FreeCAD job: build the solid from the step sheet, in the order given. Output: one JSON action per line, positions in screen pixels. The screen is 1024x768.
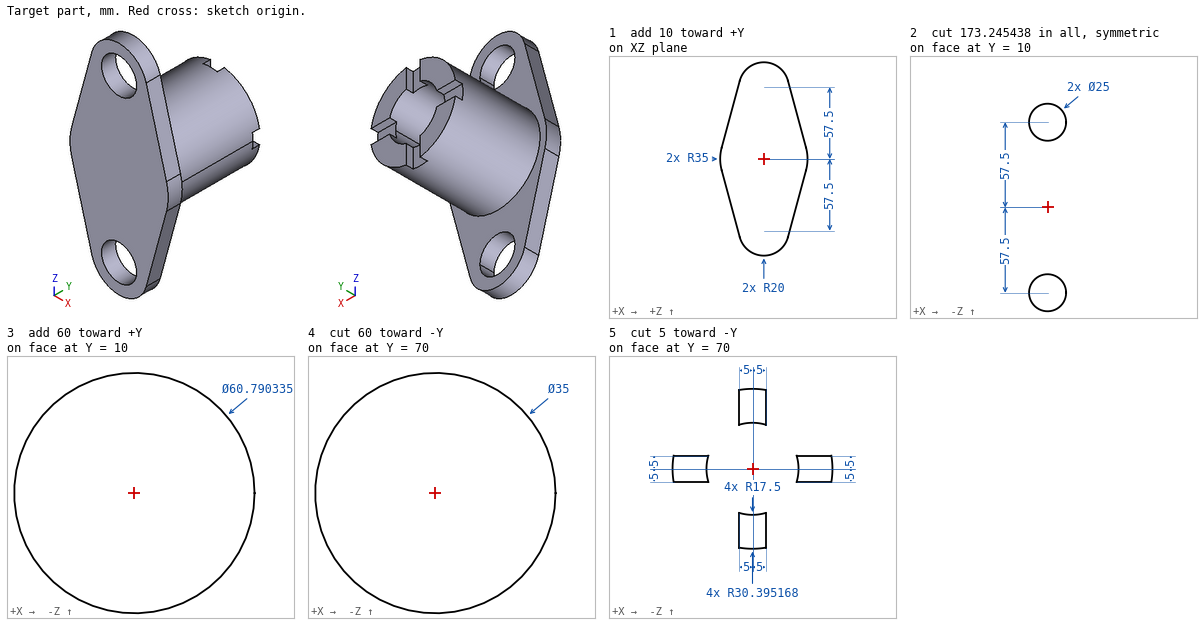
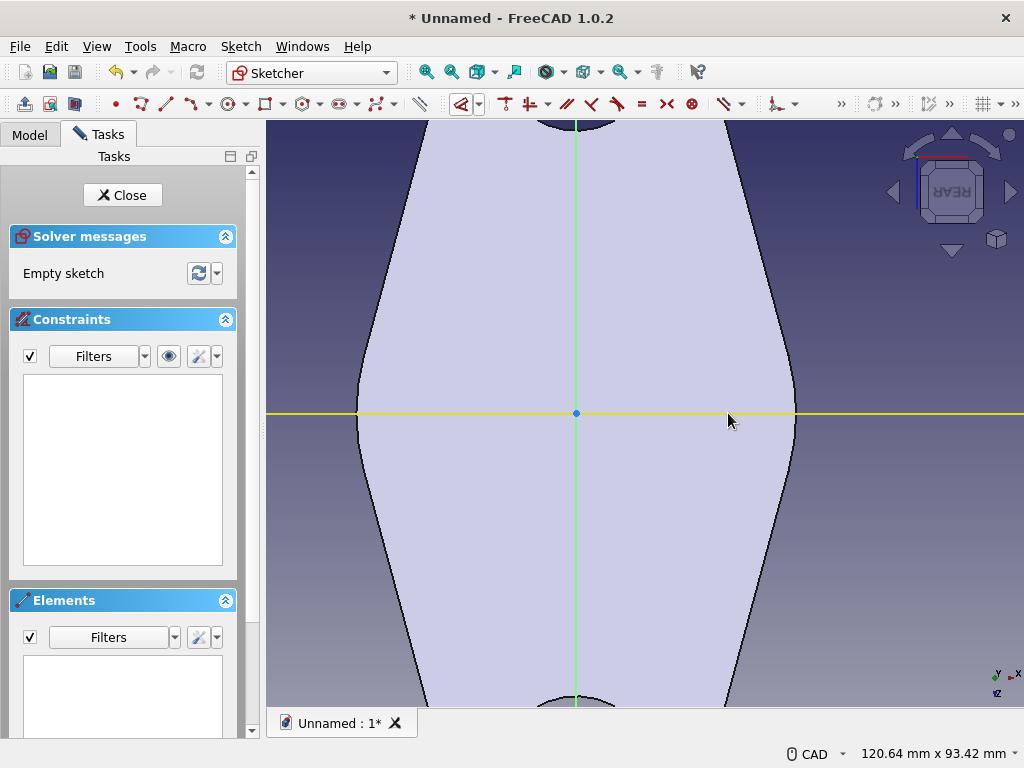
{"action": "left_click", "coordinate": [228, 104]}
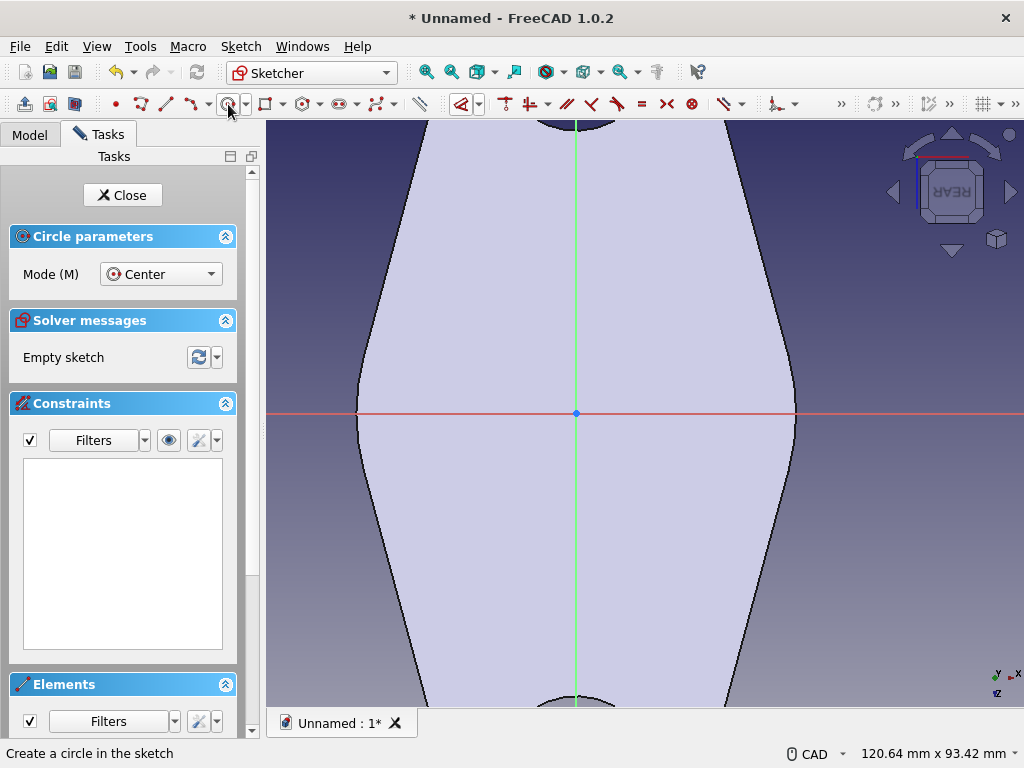
{"action": "left_click", "coordinate": [576, 413]}
{"action": "mouse_move", "coordinate": [711, 278]}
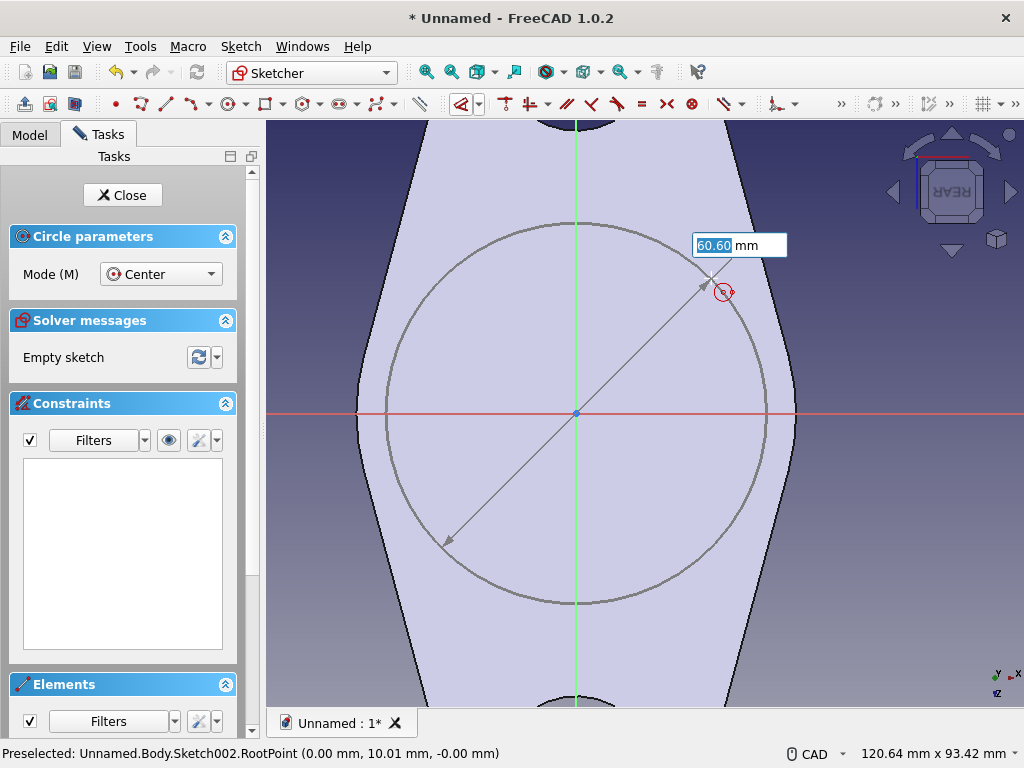
{"action": "type", "text": "60.790335"}
{"action": "key", "text": "Return"}
{"action": "key", "text": "Escape"}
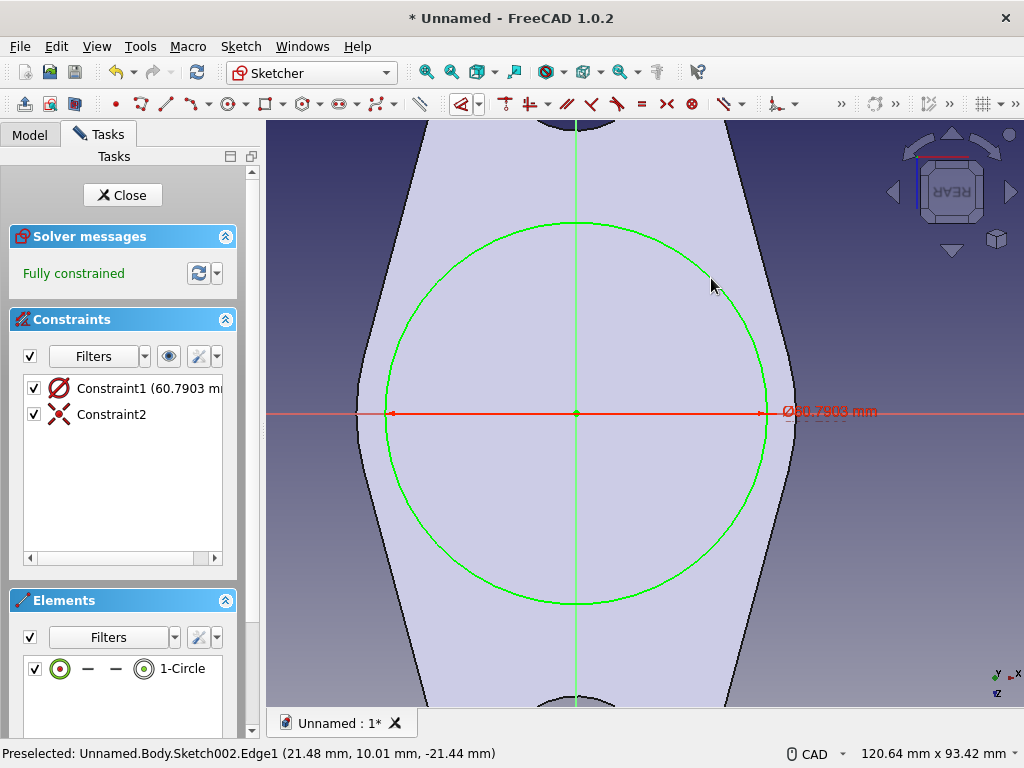
{"action": "left_click", "coordinate": [123, 195]}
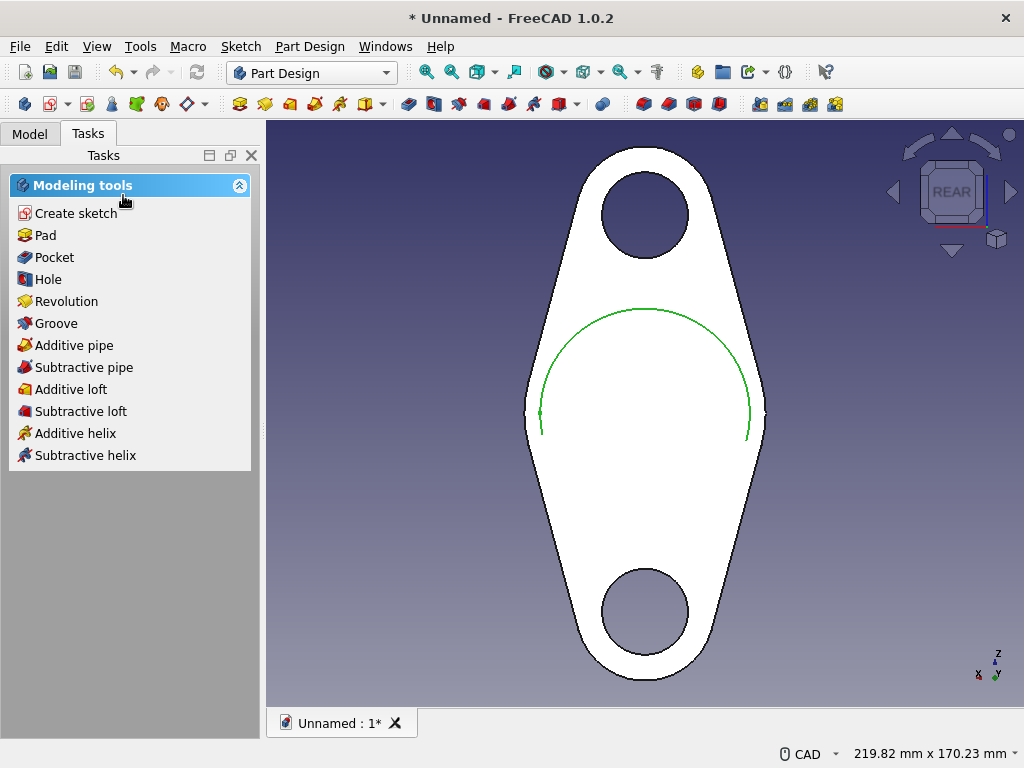
{"action": "left_click", "coordinate": [240, 104]}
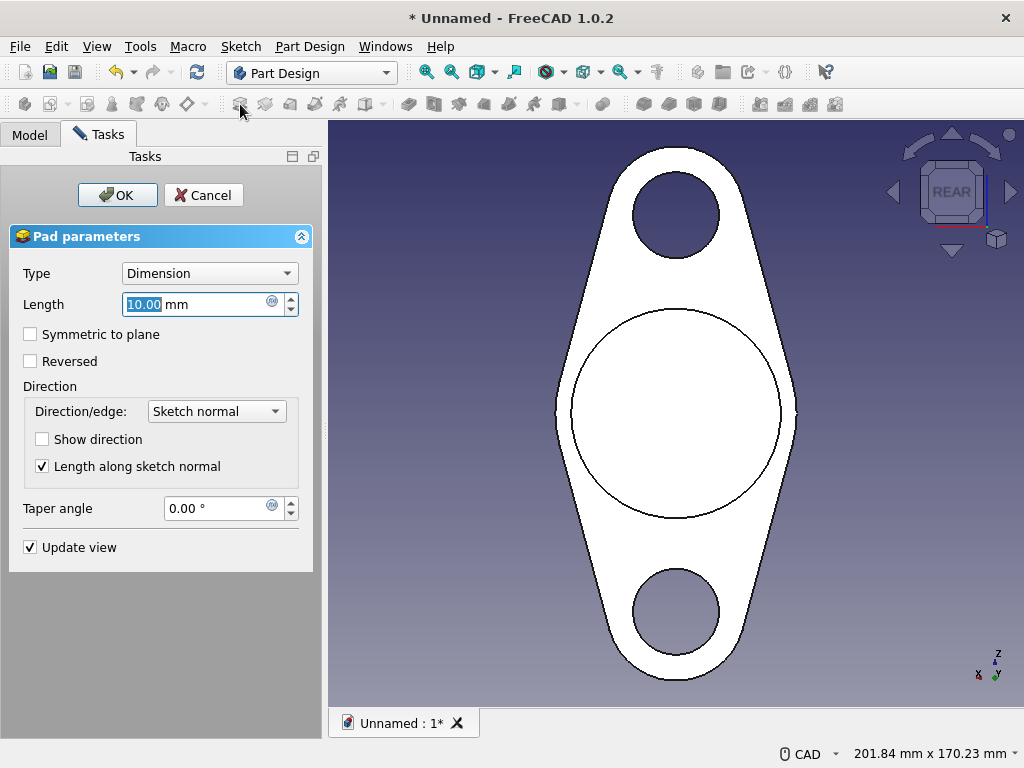
{"action": "type", "text": "60"}
{"action": "key", "text": "Tab"}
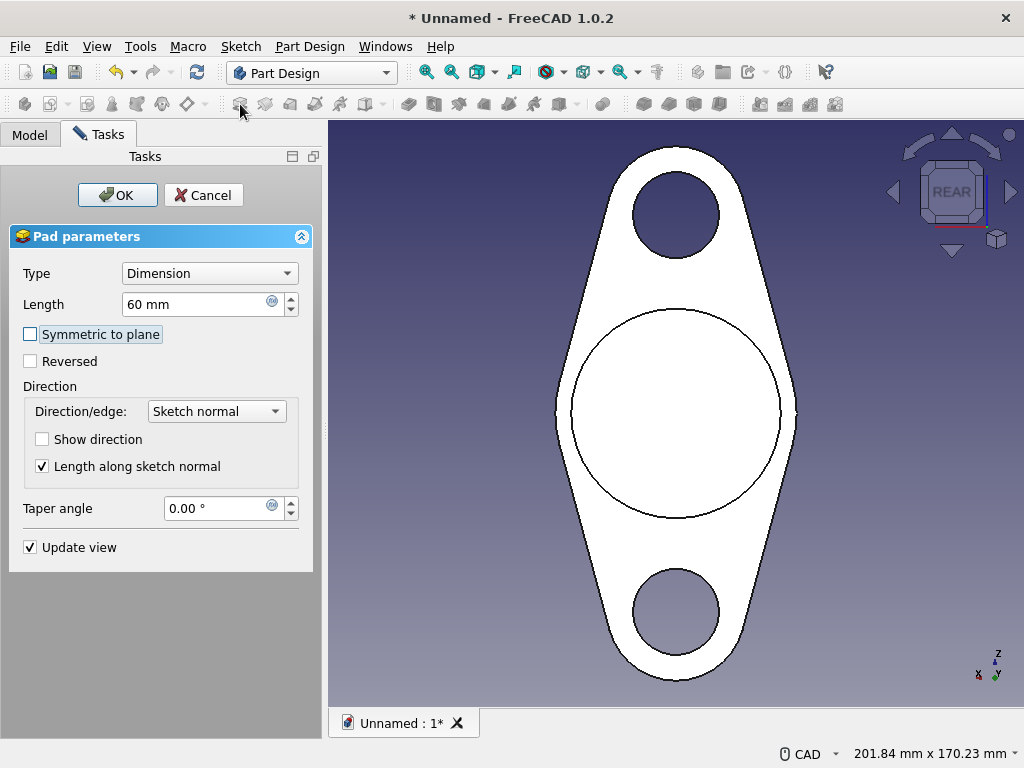
{"action": "left_click", "coordinate": [118, 195]}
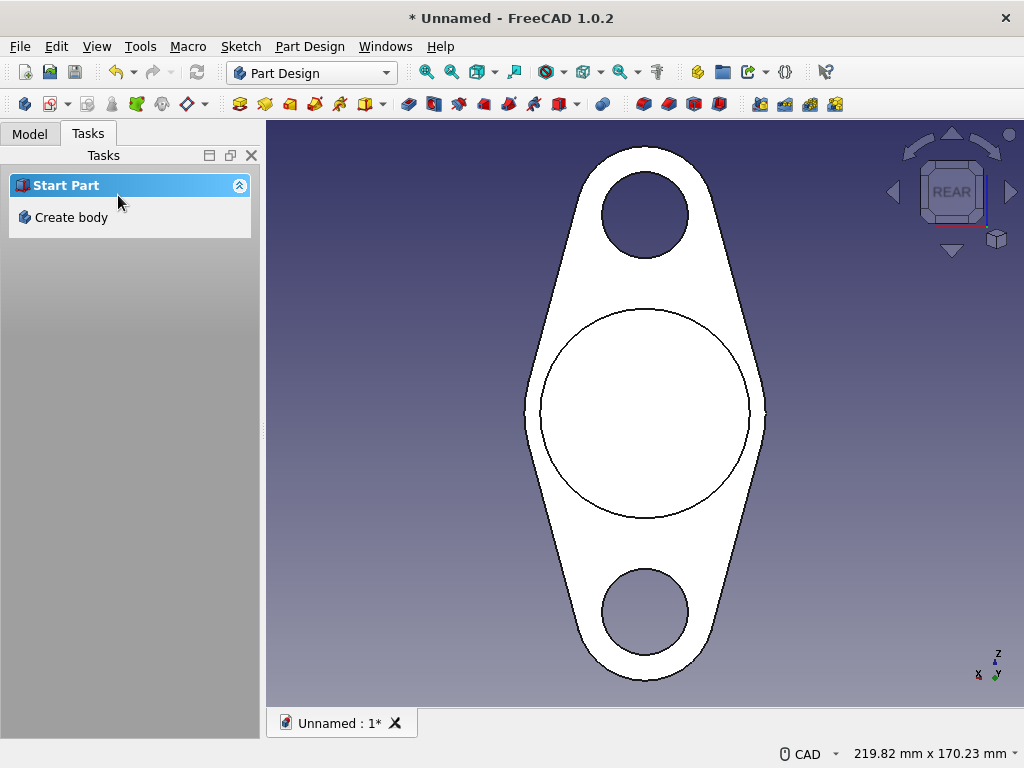
{"action": "left_click", "coordinate": [645, 412]}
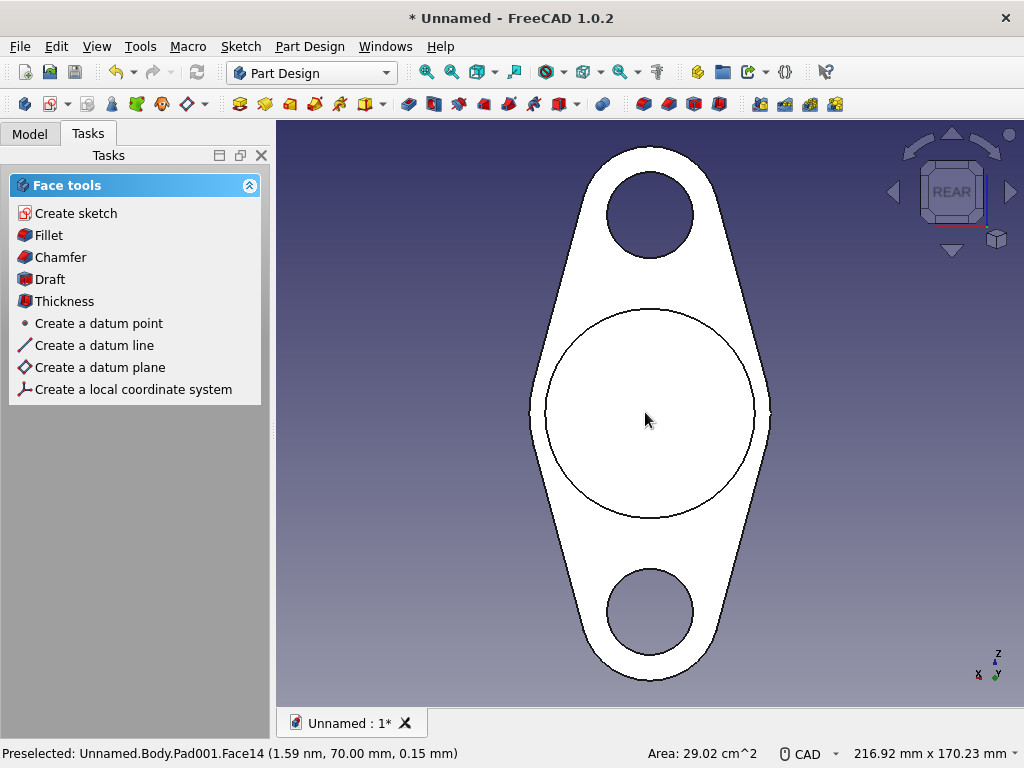
{"action": "left_click", "coordinate": [50, 104]}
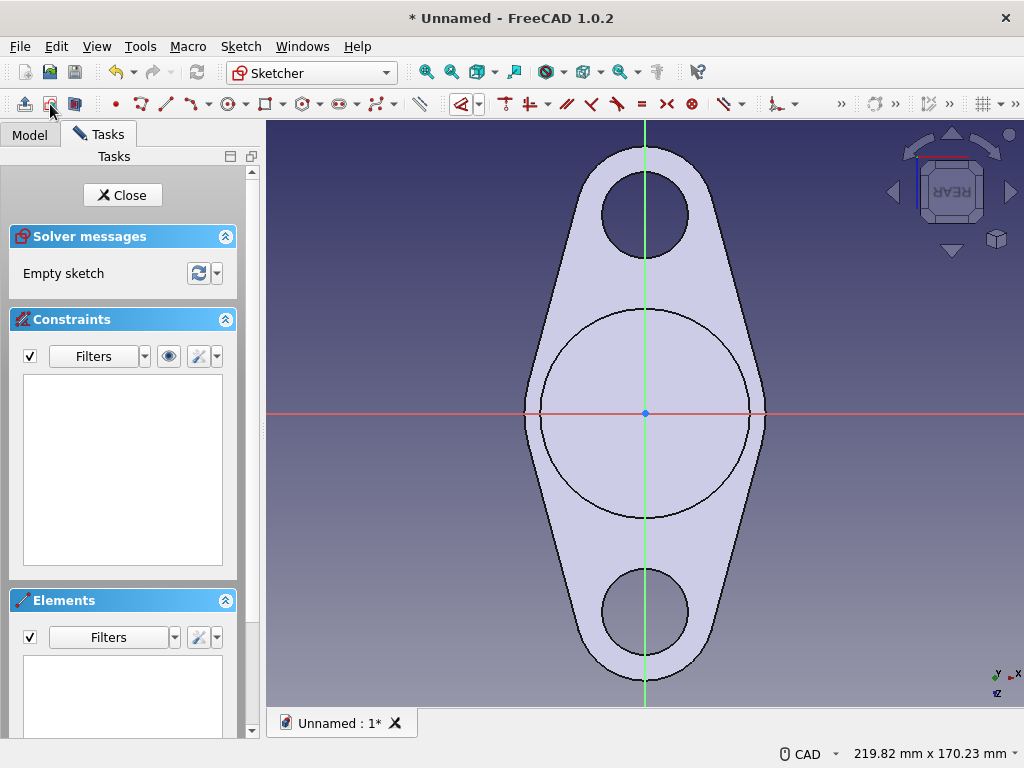
{"action": "scroll", "coordinate": [675, 413], "scroll_direction": "up", "scroll_amount": 6}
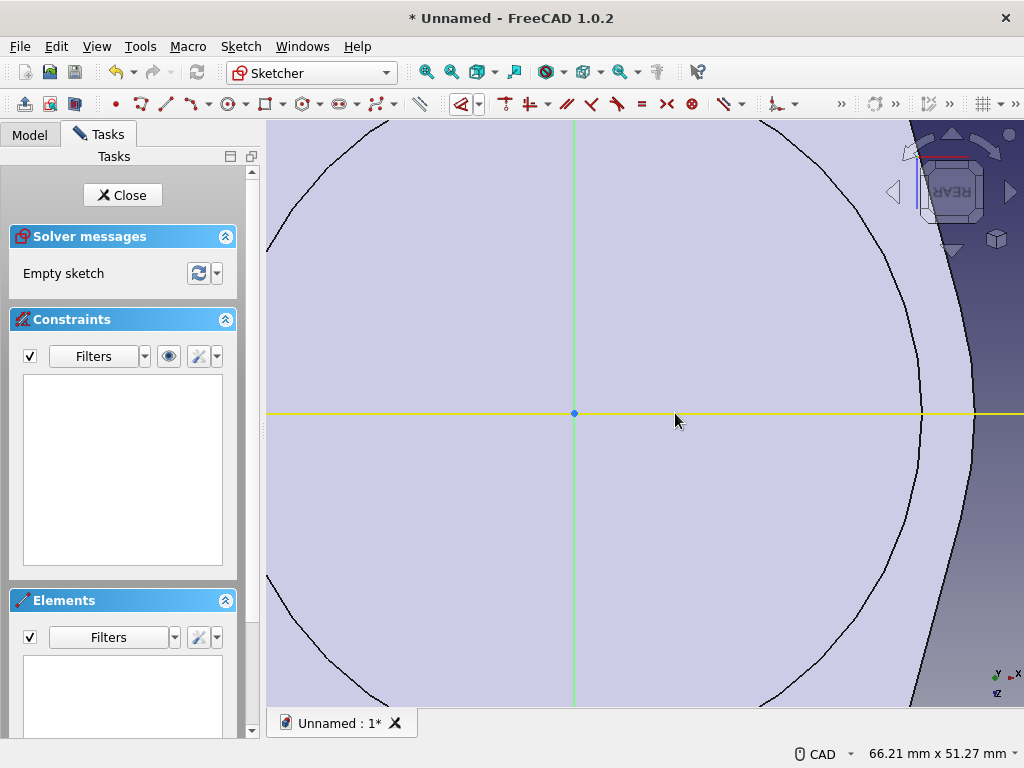
{"action": "left_click", "coordinate": [228, 104]}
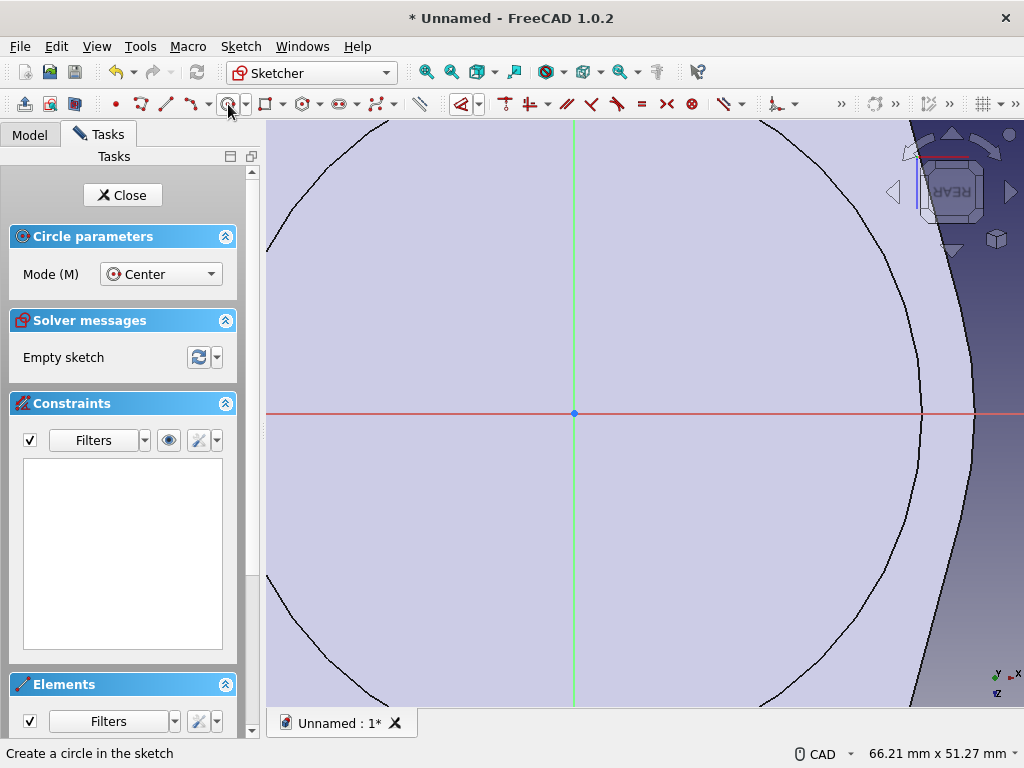
{"action": "left_click", "coordinate": [574, 413]}
{"action": "mouse_move", "coordinate": [716, 272]}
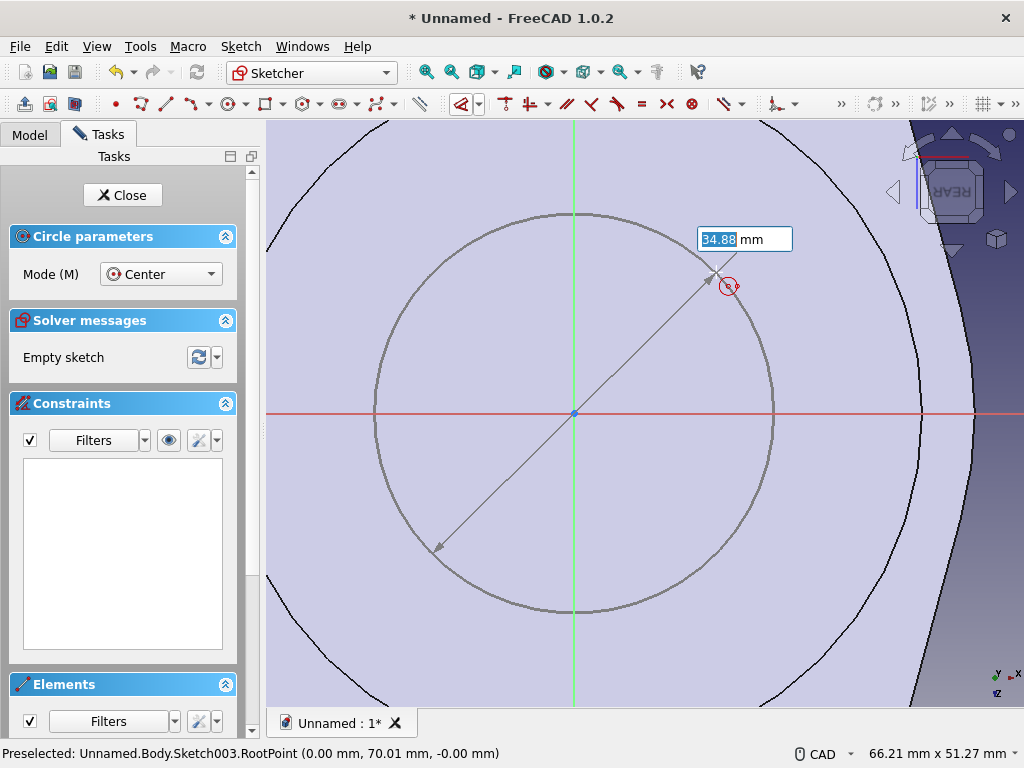
{"action": "type", "text": "35"}
{"action": "key", "text": "Return"}
{"action": "key", "text": "Escape"}